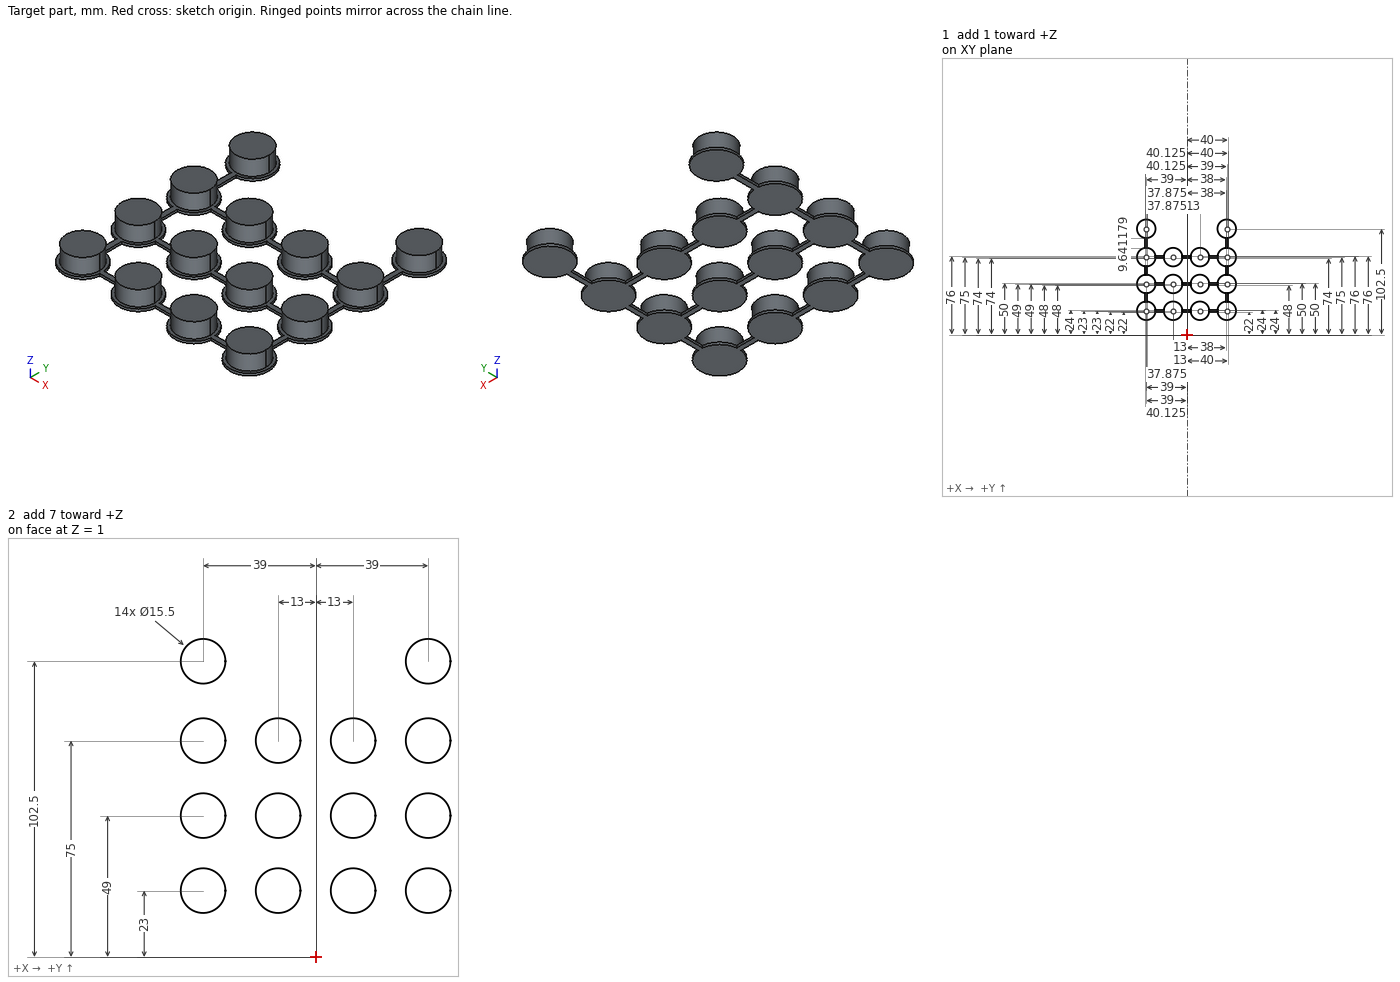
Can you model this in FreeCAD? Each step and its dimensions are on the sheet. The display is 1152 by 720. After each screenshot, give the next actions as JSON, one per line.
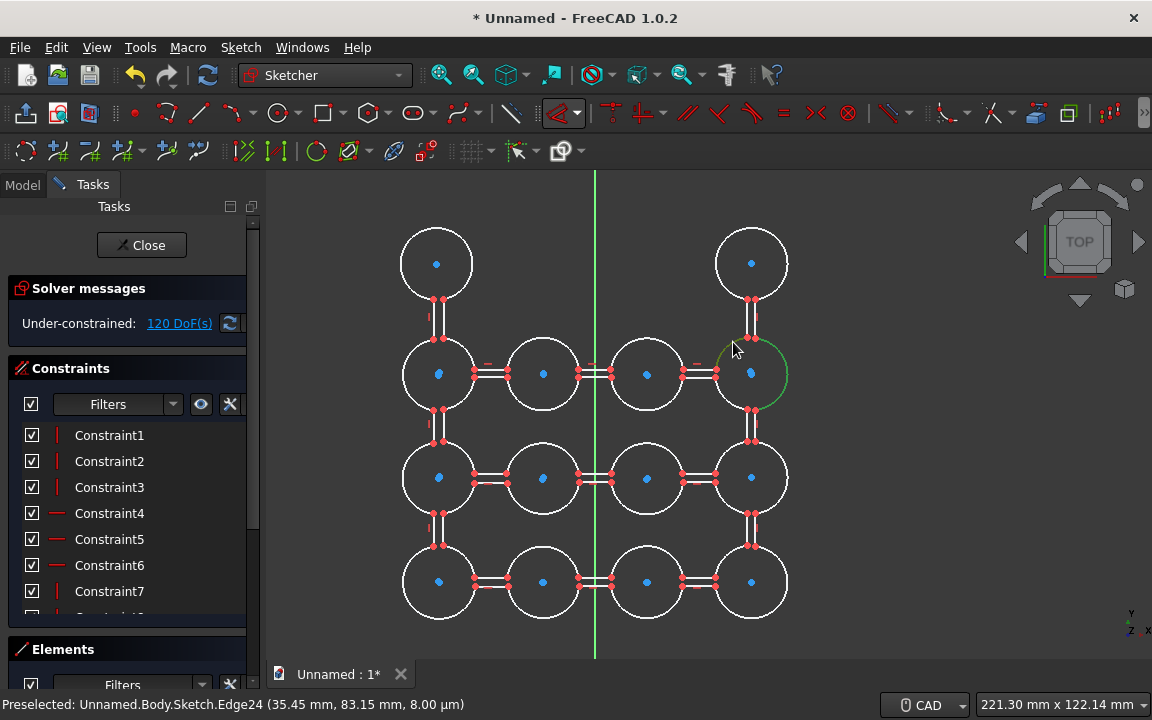
{"action": "left_click", "coordinate": [612, 114]}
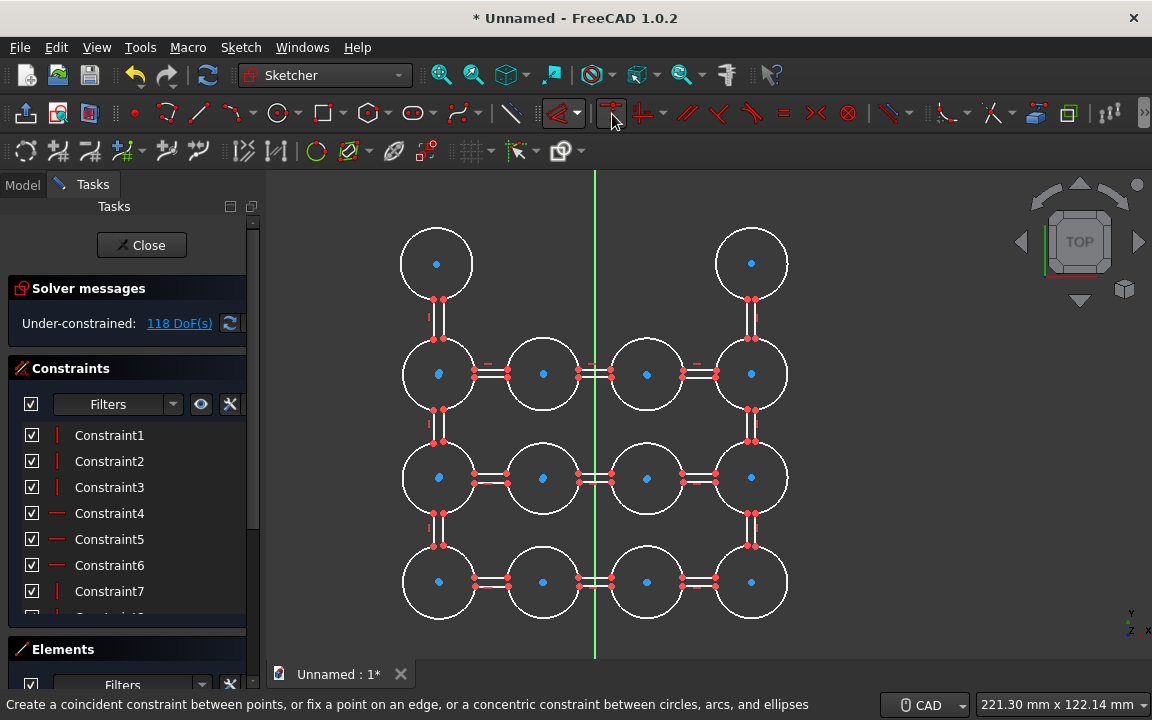
{"action": "left_click", "coordinate": [409, 356]}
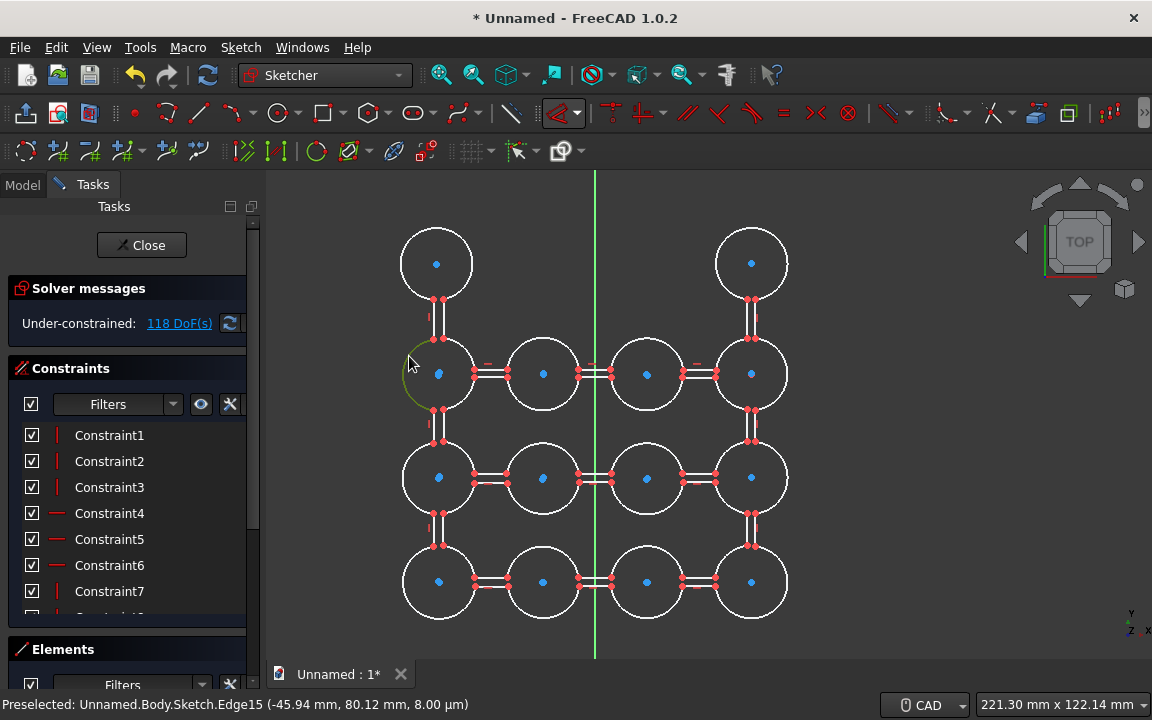
{"action": "left_click", "coordinate": [470, 356]}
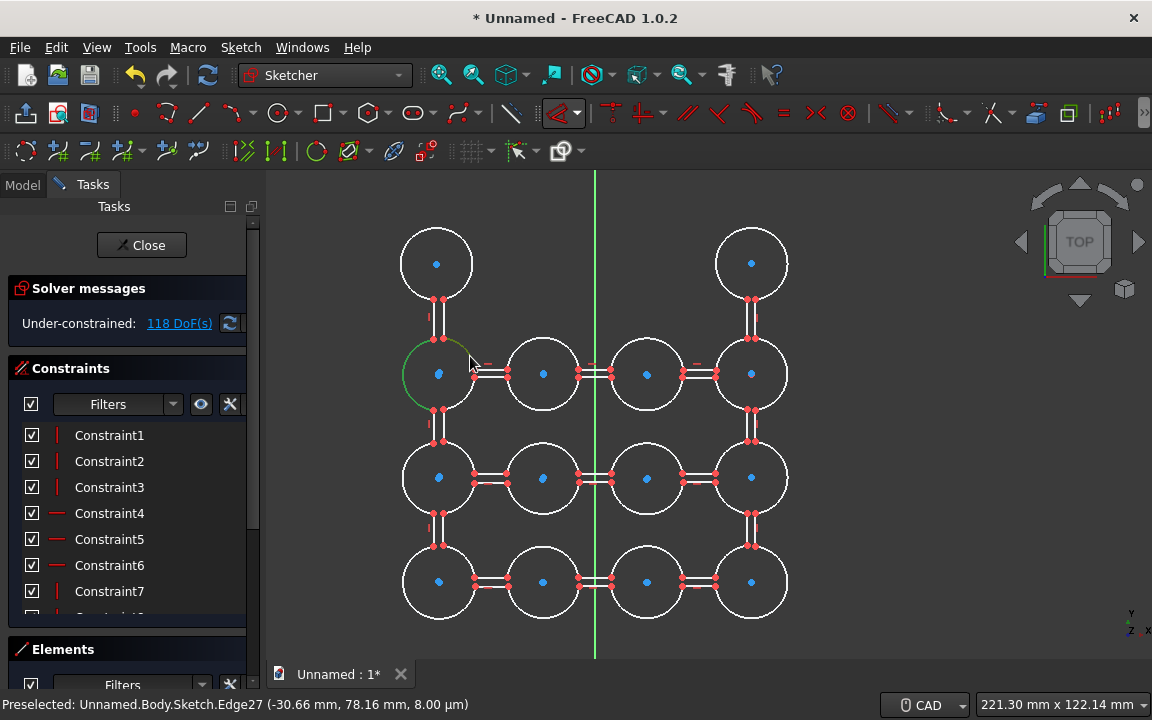
{"action": "left_click", "coordinate": [612, 114]}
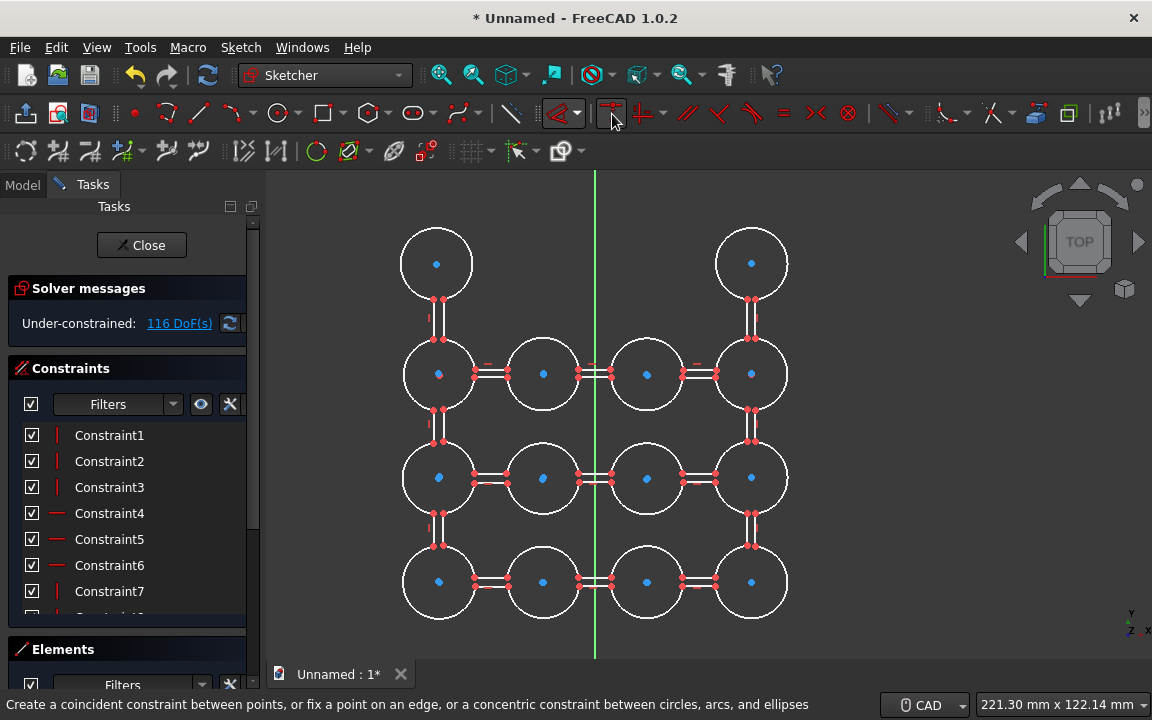
{"action": "left_click", "coordinate": [782, 498]}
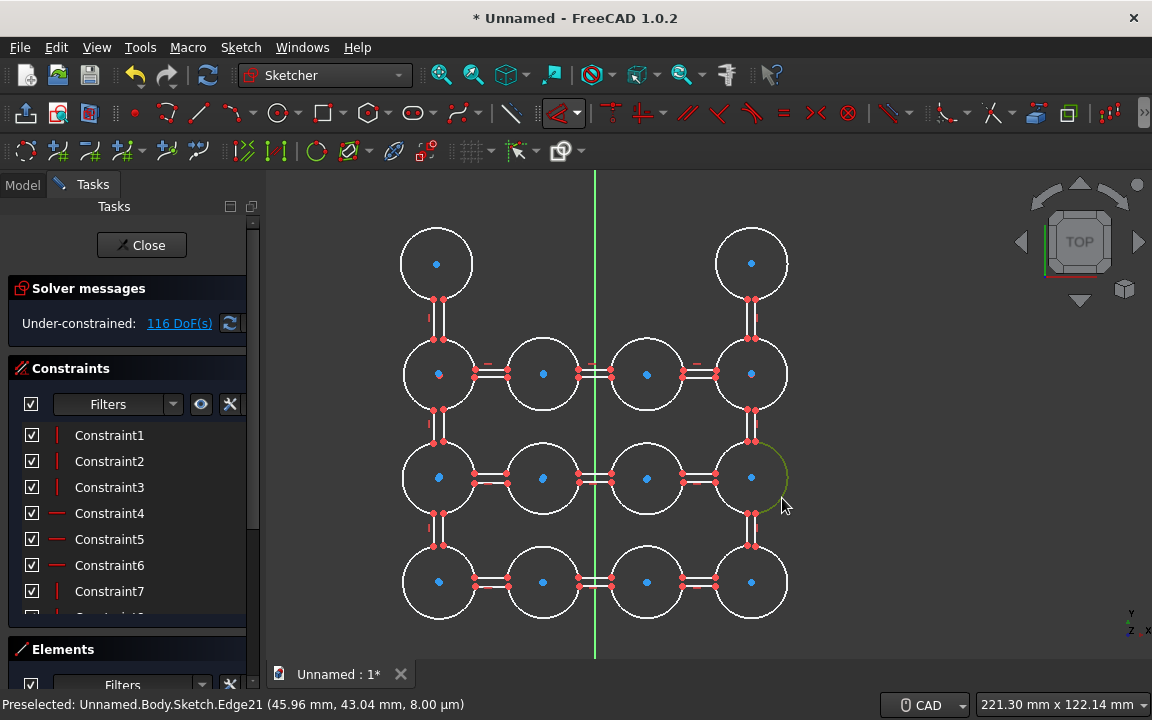
{"action": "left_click", "coordinate": [720, 496]}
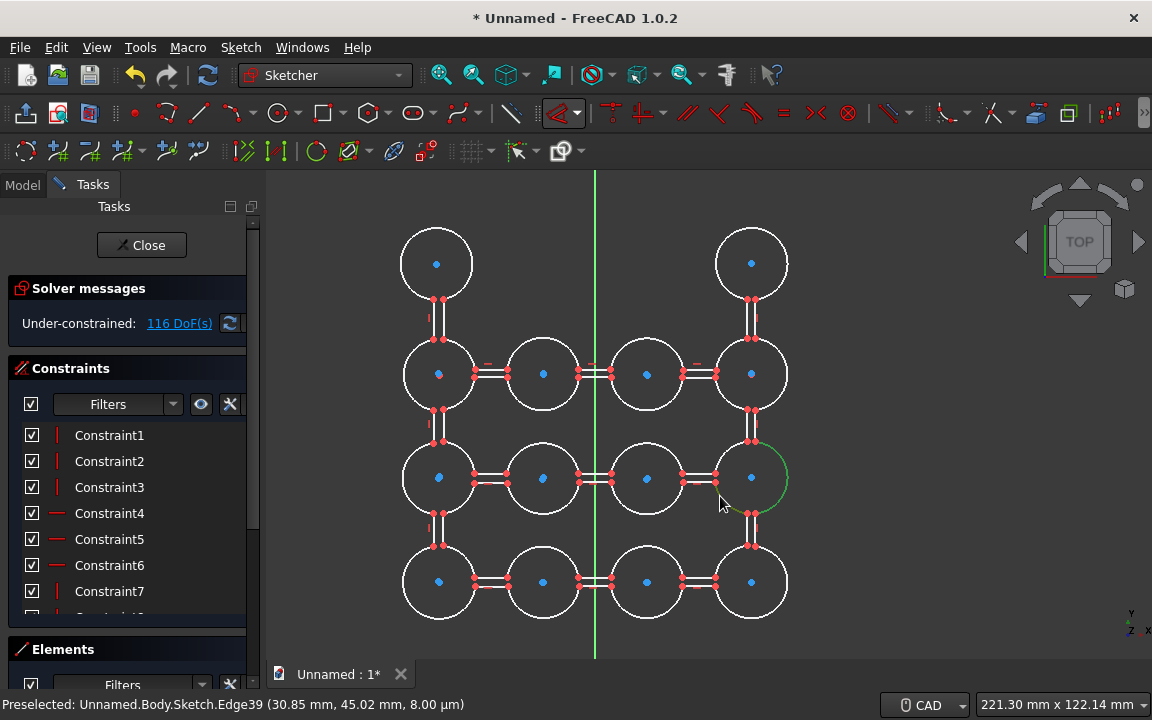
{"action": "left_click", "coordinate": [612, 114]}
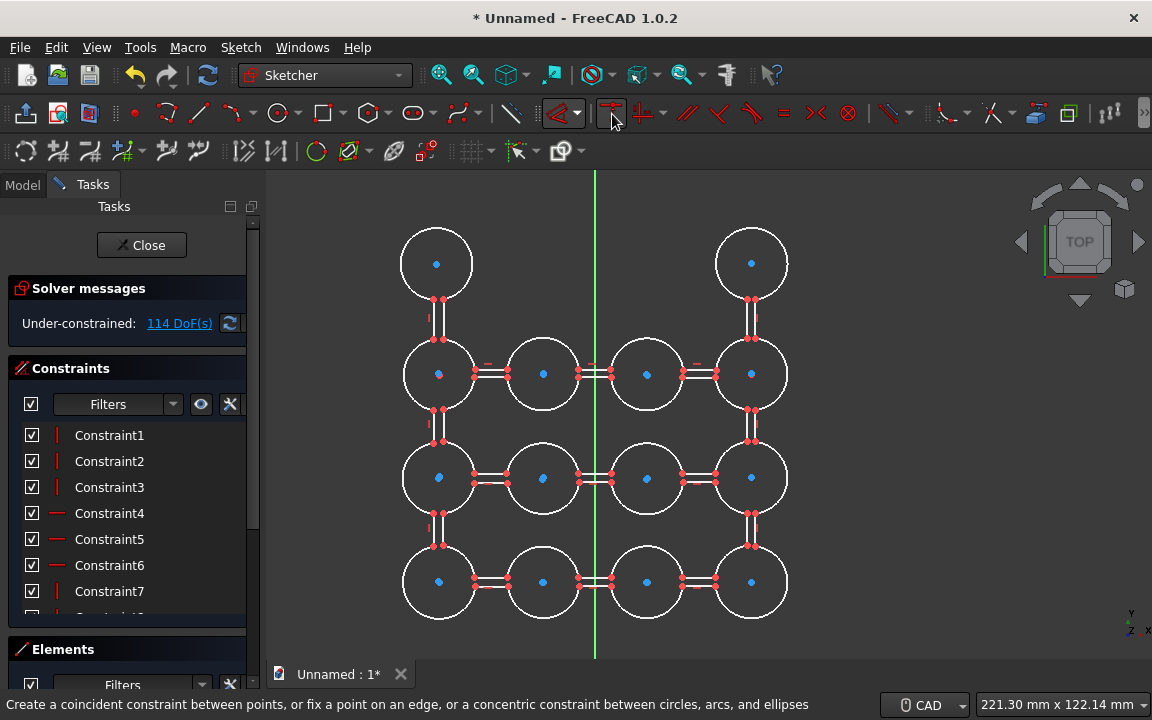
{"action": "left_click", "coordinate": [747, 618]}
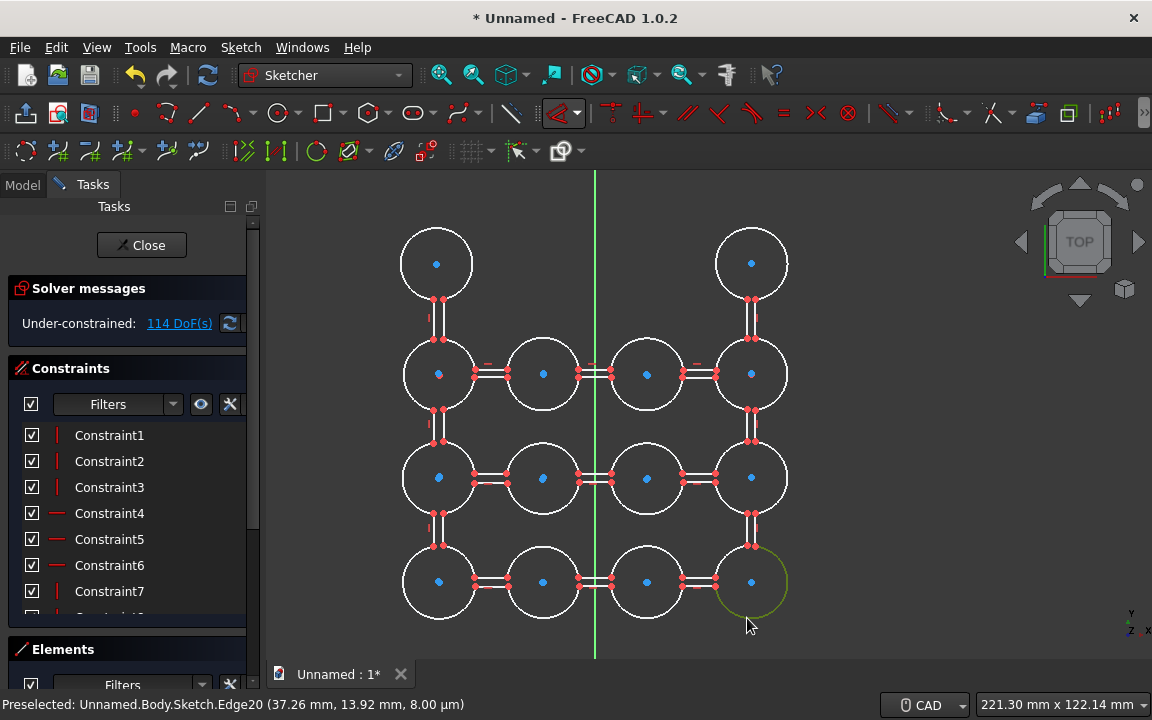
{"action": "left_click", "coordinate": [733, 550]}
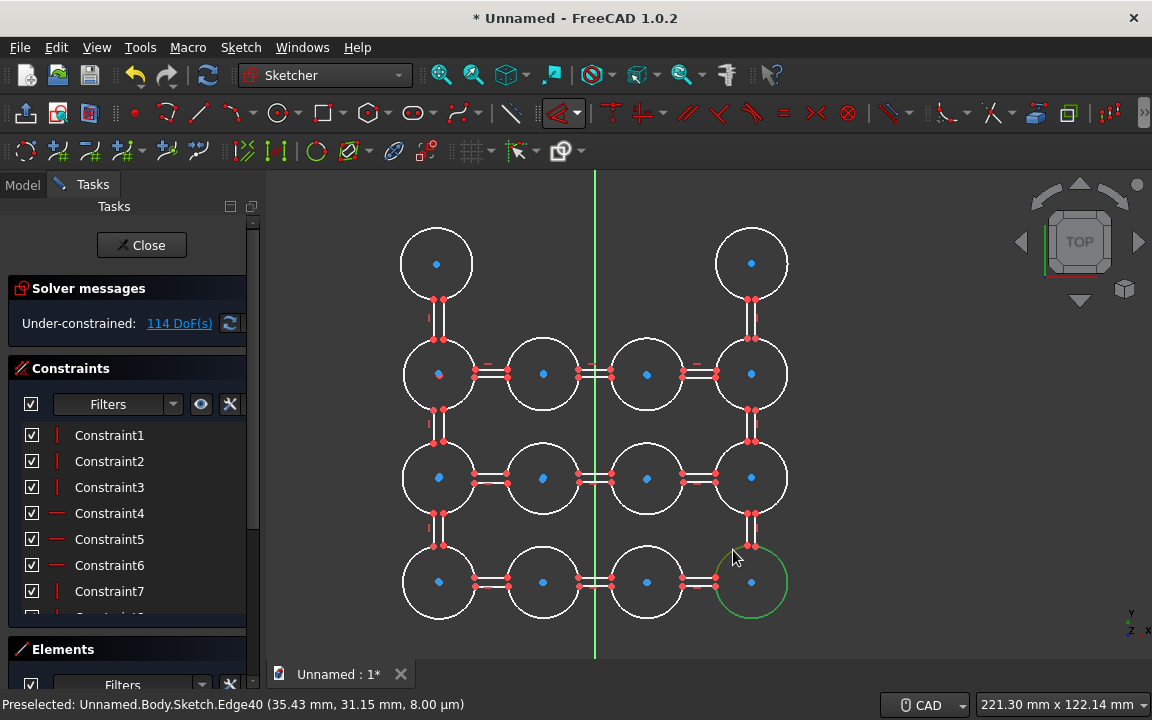
{"action": "left_click", "coordinate": [612, 114]}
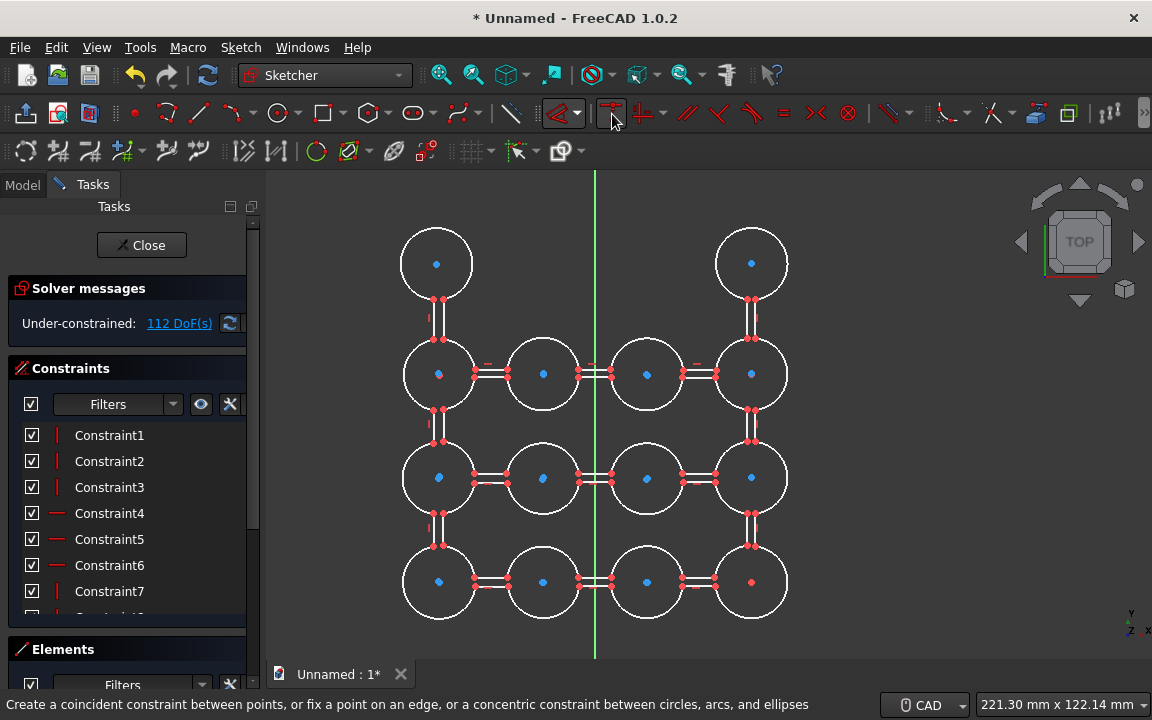
{"action": "left_click", "coordinate": [627, 612]}